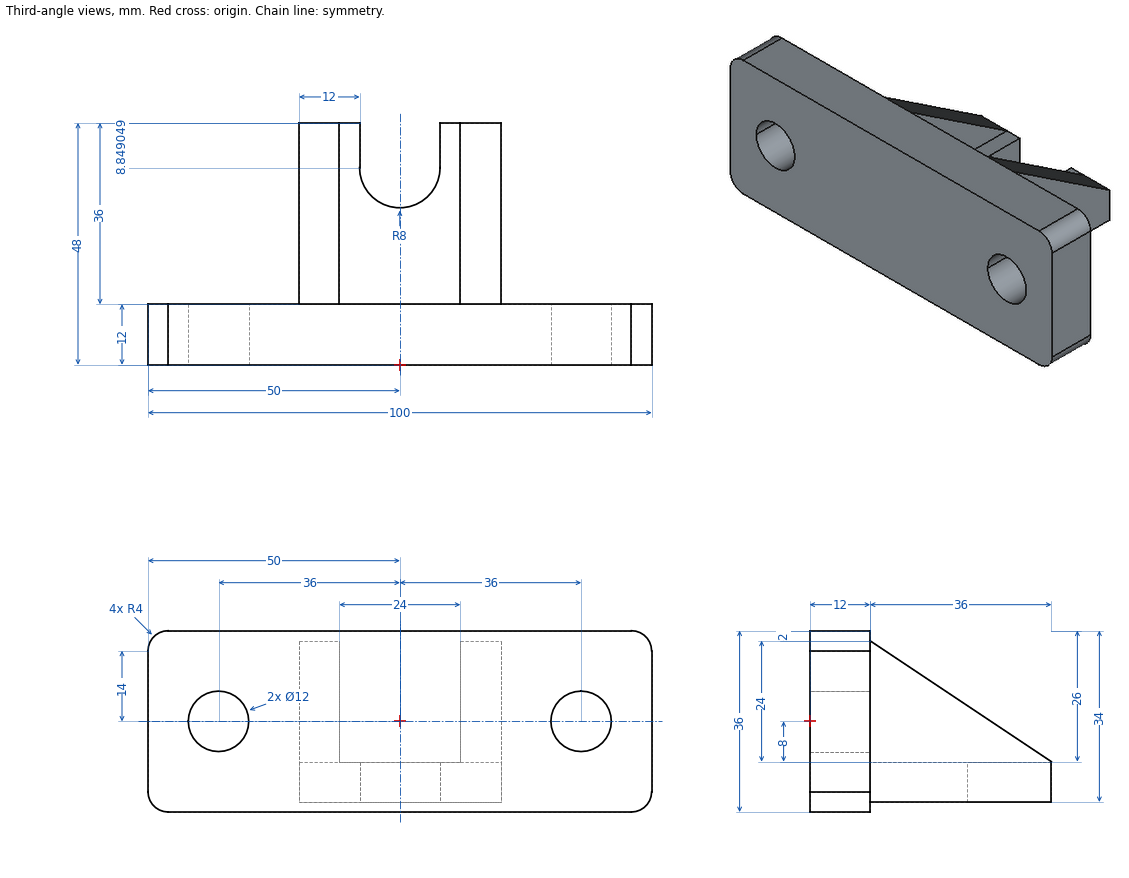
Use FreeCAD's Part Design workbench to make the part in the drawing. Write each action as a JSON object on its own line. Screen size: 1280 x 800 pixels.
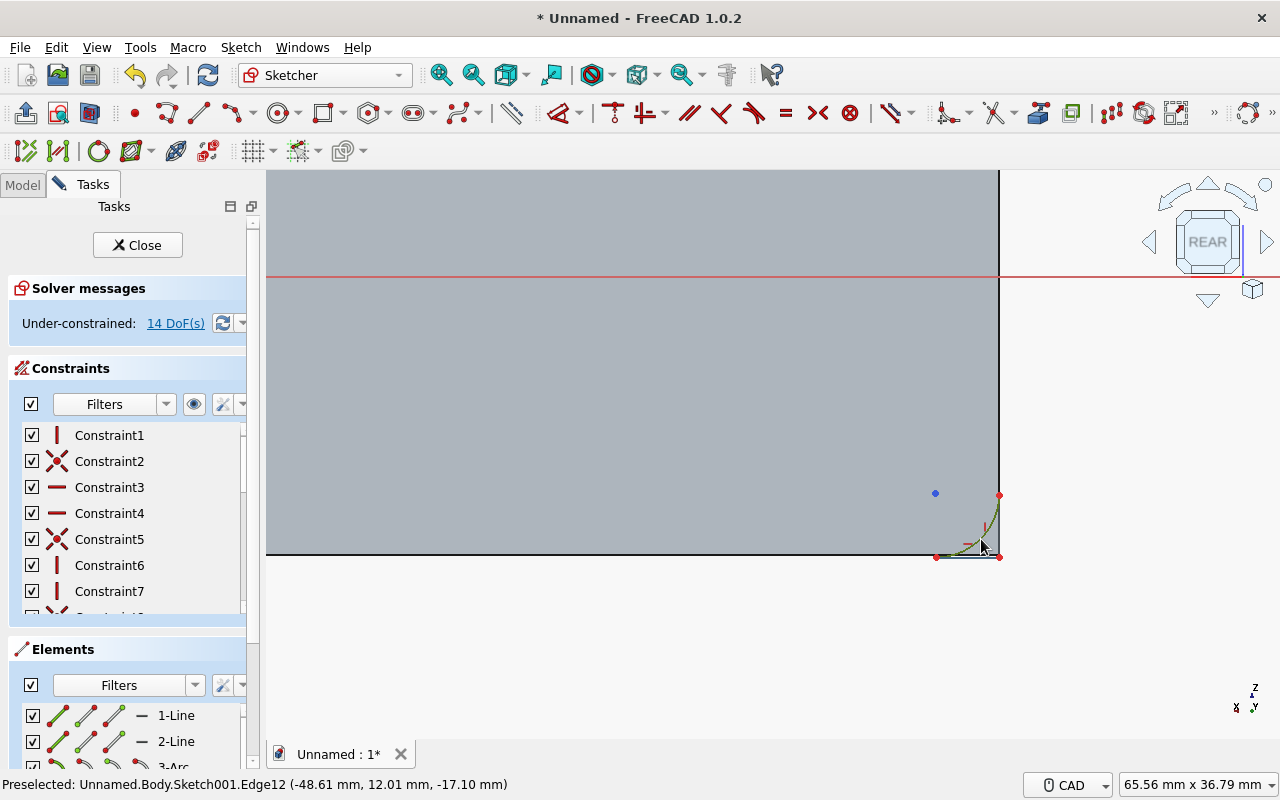
{"action": "left_click", "coordinate": [754, 114]}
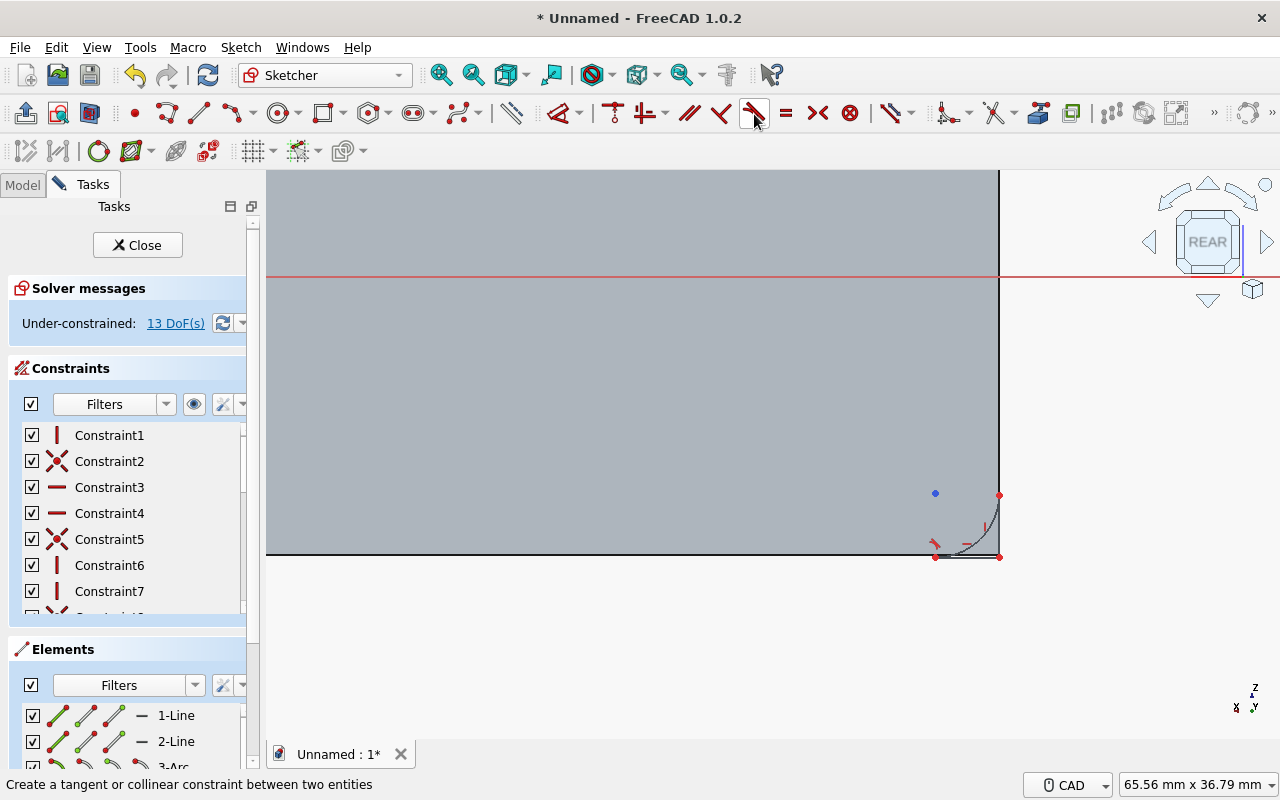
{"action": "left_click", "coordinate": [999, 539]}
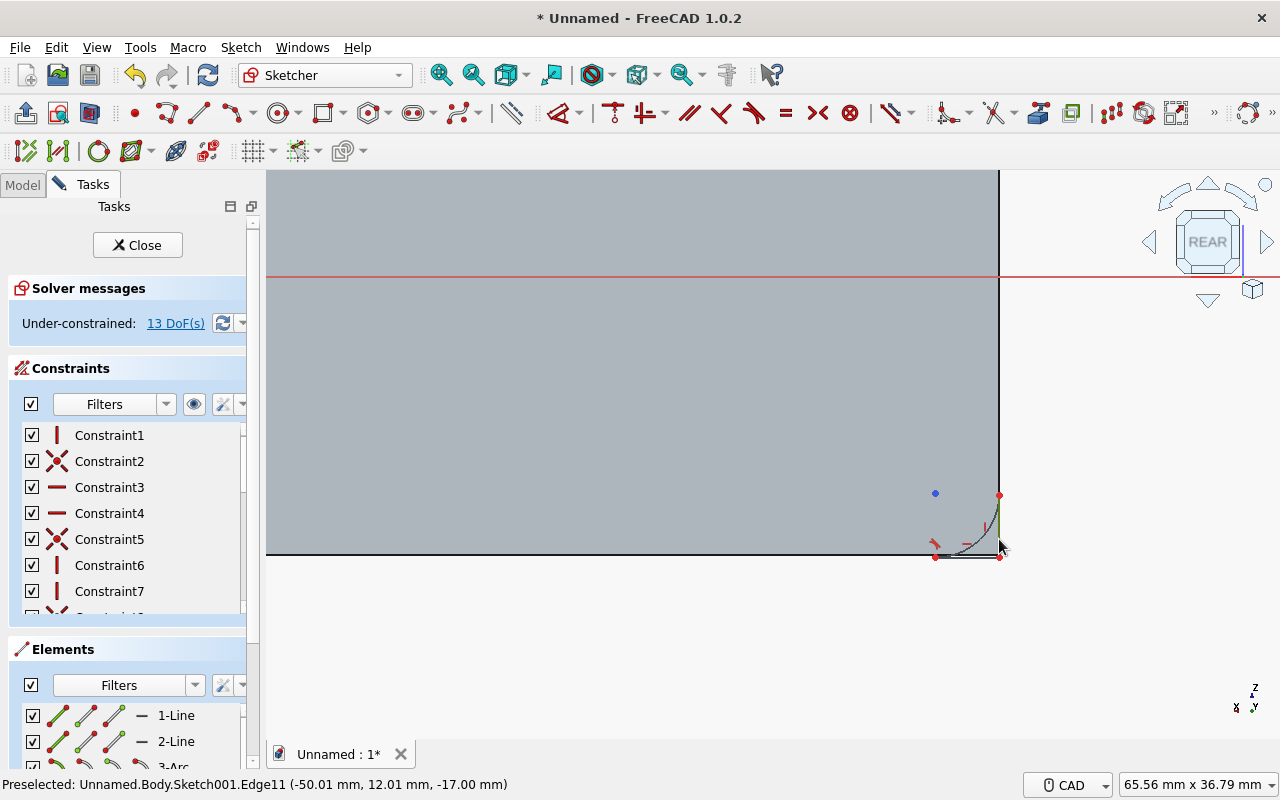
{"action": "left_click", "coordinate": [980, 539]}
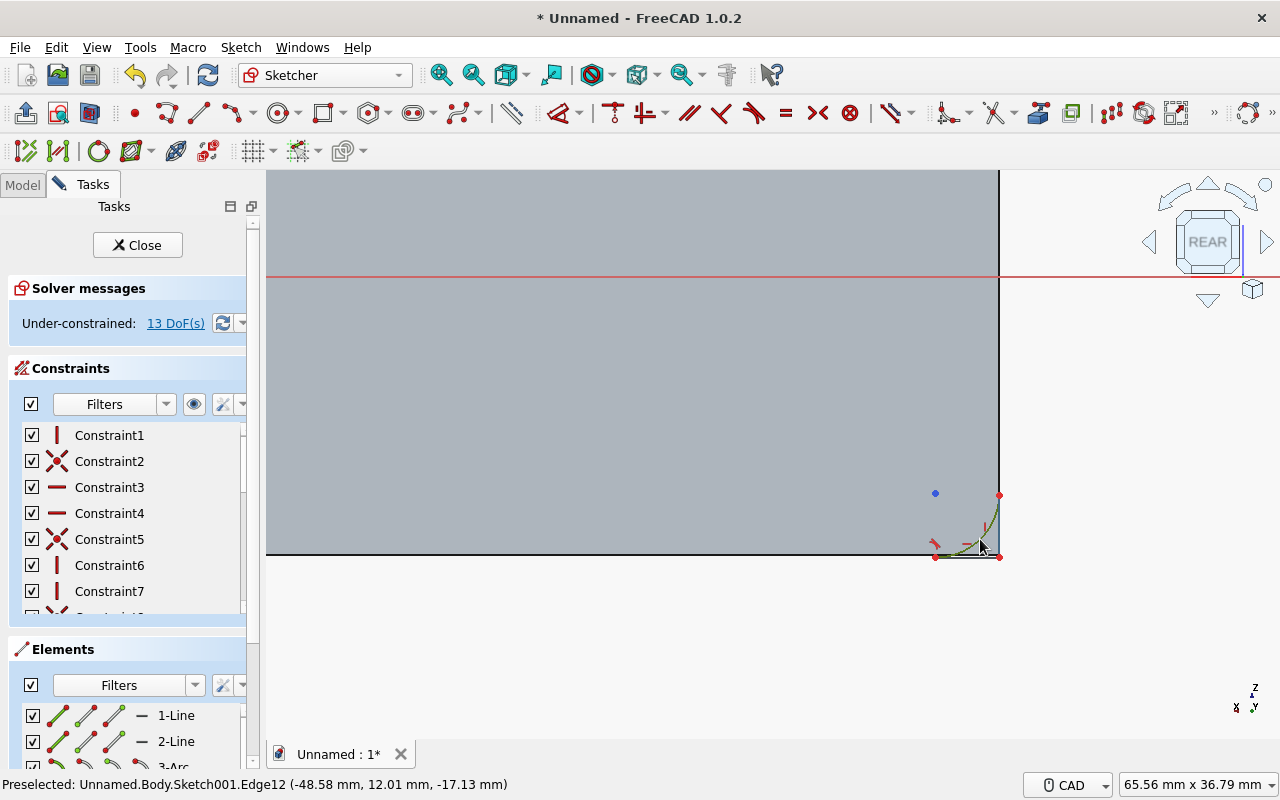
{"action": "left_click", "coordinate": [754, 114]}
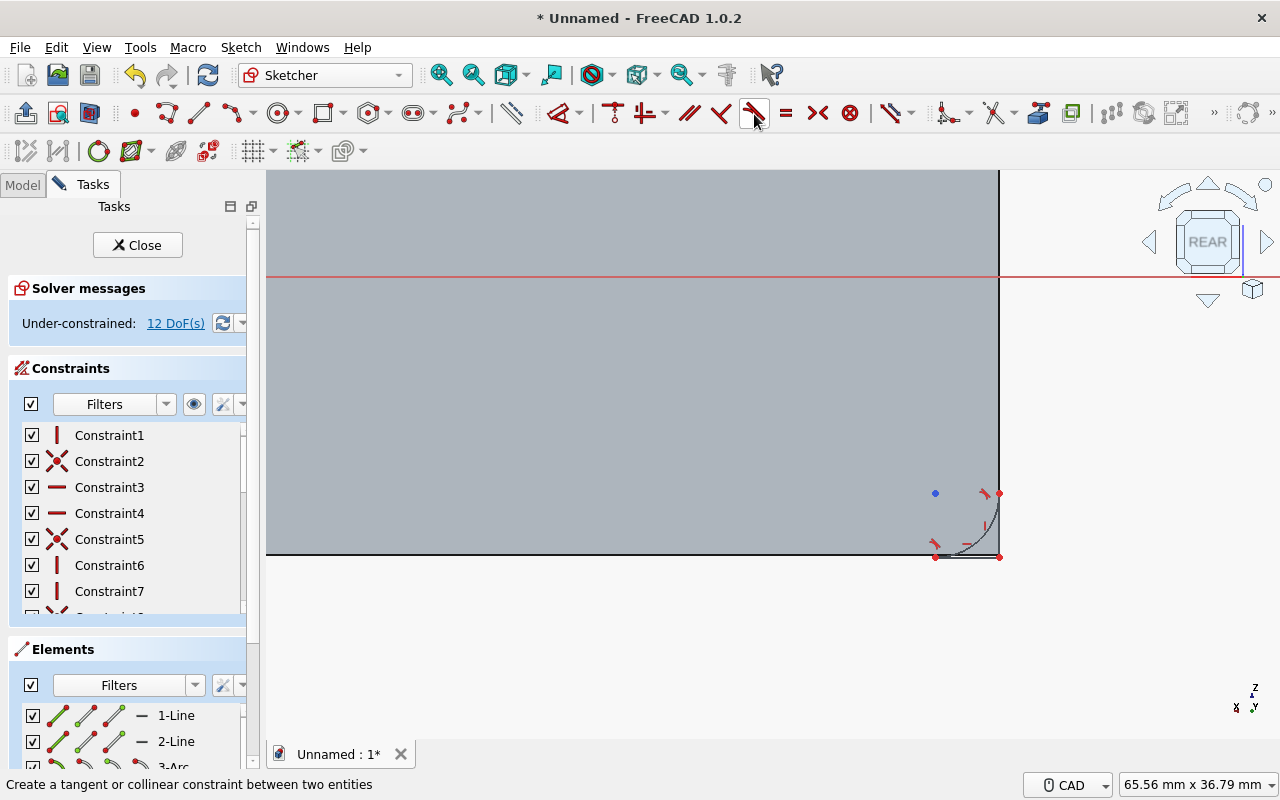
{"action": "scroll", "coordinate": [983, 558], "scroll_direction": "down", "scroll_amount": 5}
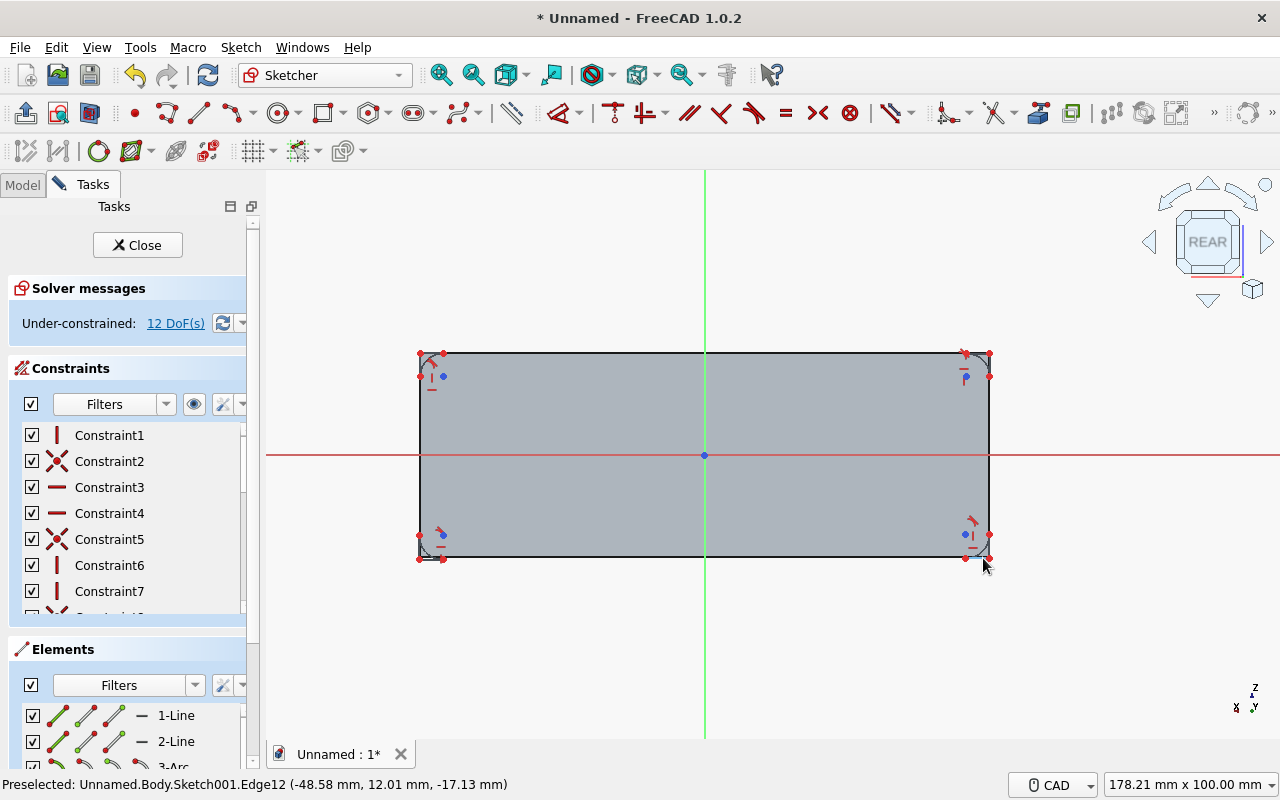
{"action": "scroll", "coordinate": [983, 360], "scroll_direction": "up", "scroll_amount": 4}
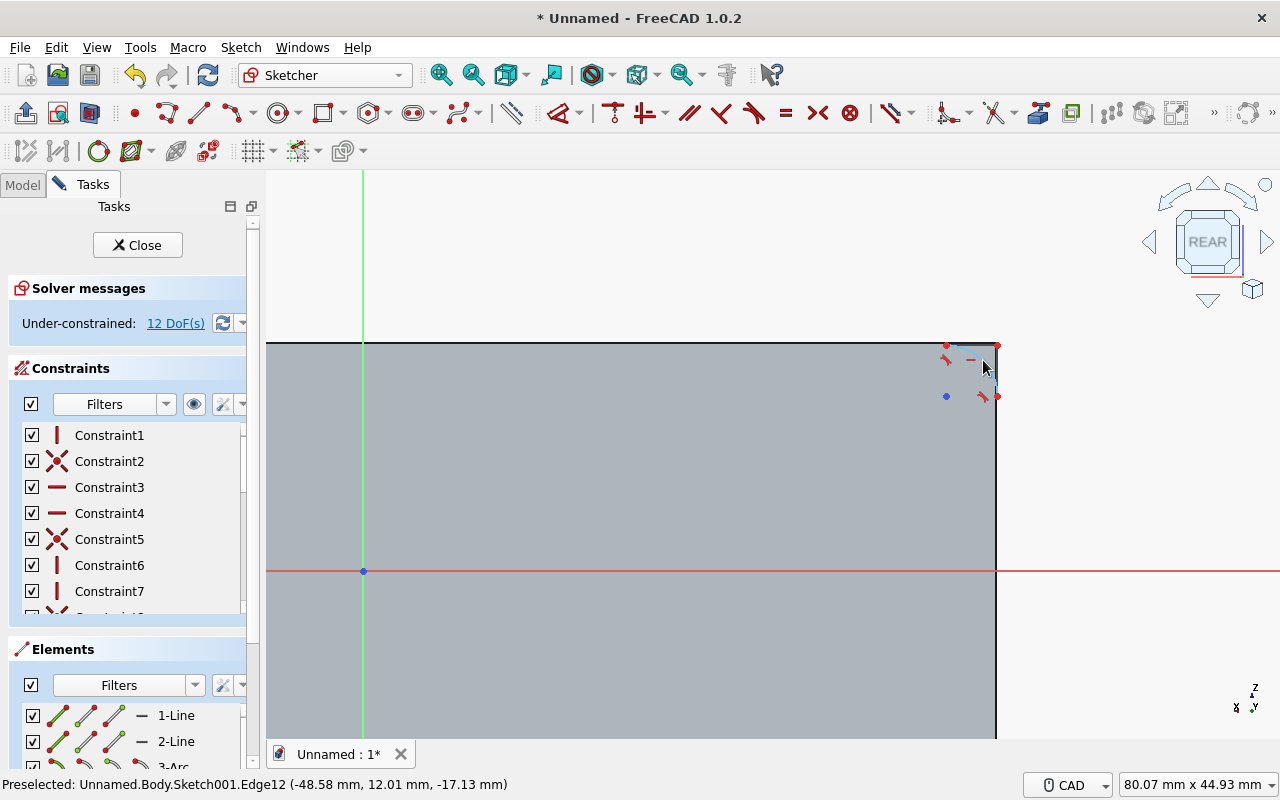
{"action": "left_click", "coordinate": [982, 360]}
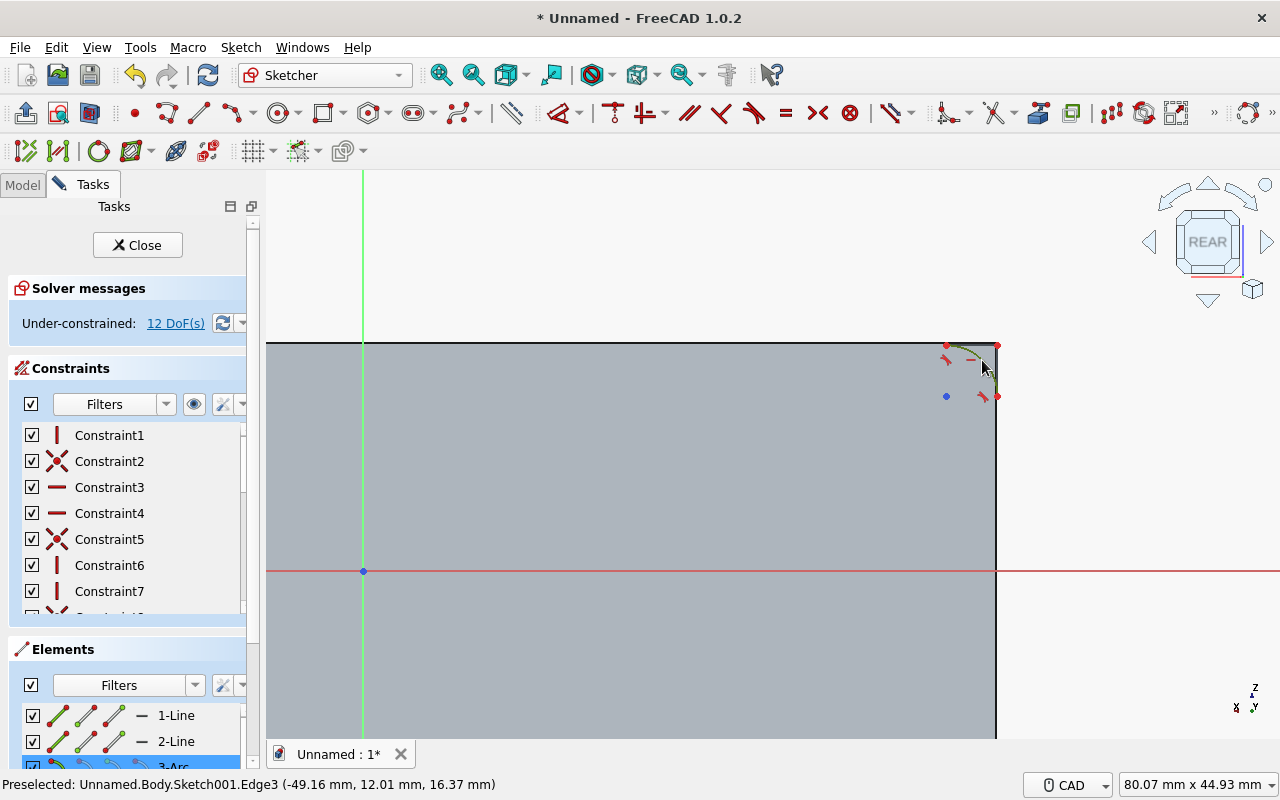
{"action": "scroll", "coordinate": [983, 359], "scroll_direction": "down", "scroll_amount": 4}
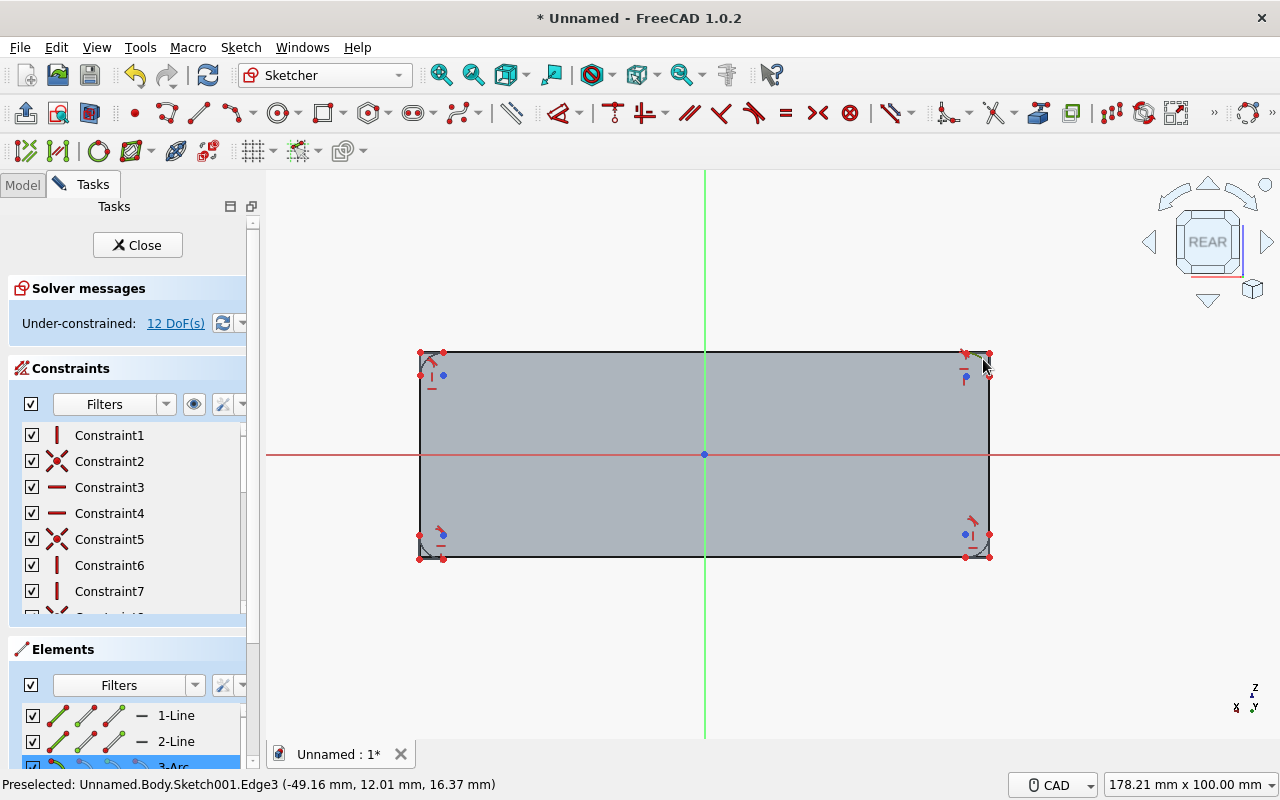
{"action": "scroll", "coordinate": [427, 360], "scroll_direction": "up", "scroll_amount": 4}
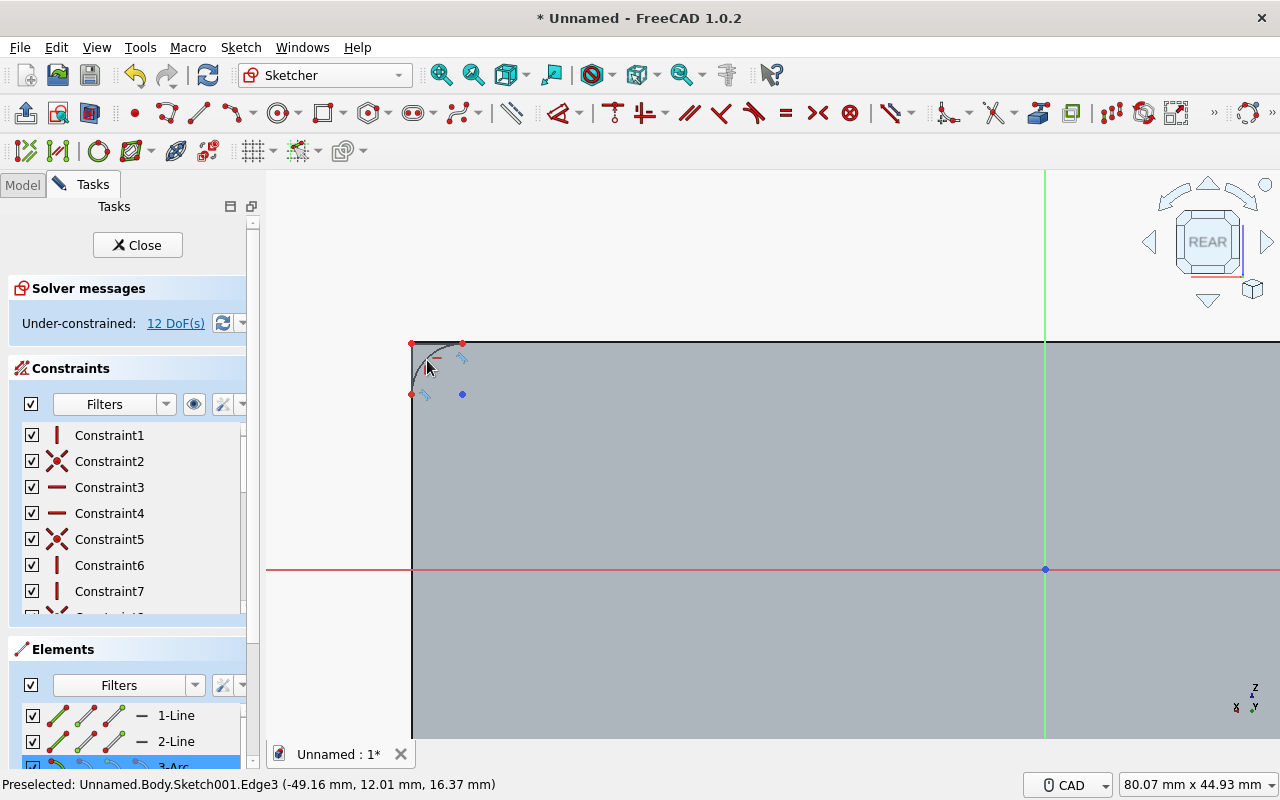
{"action": "left_click", "coordinate": [427, 359]}